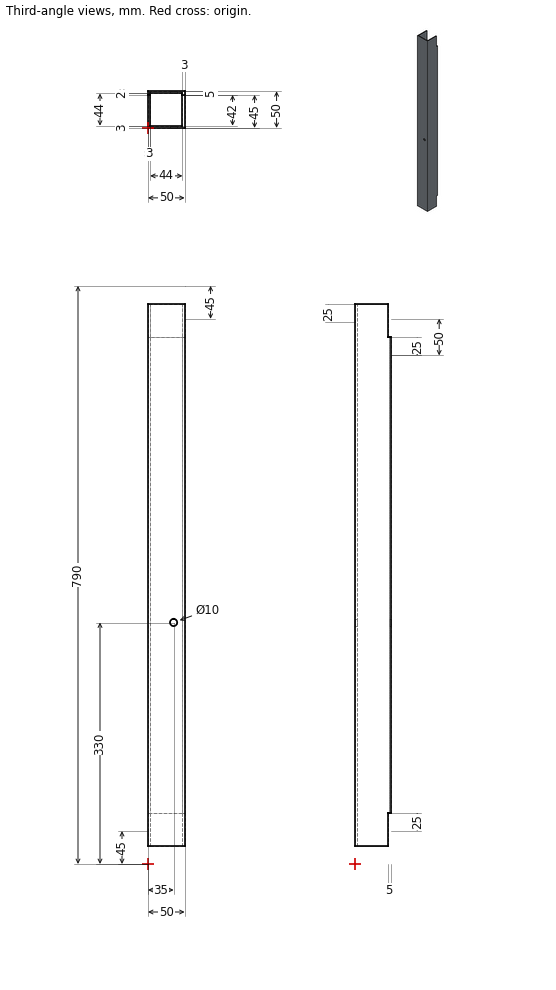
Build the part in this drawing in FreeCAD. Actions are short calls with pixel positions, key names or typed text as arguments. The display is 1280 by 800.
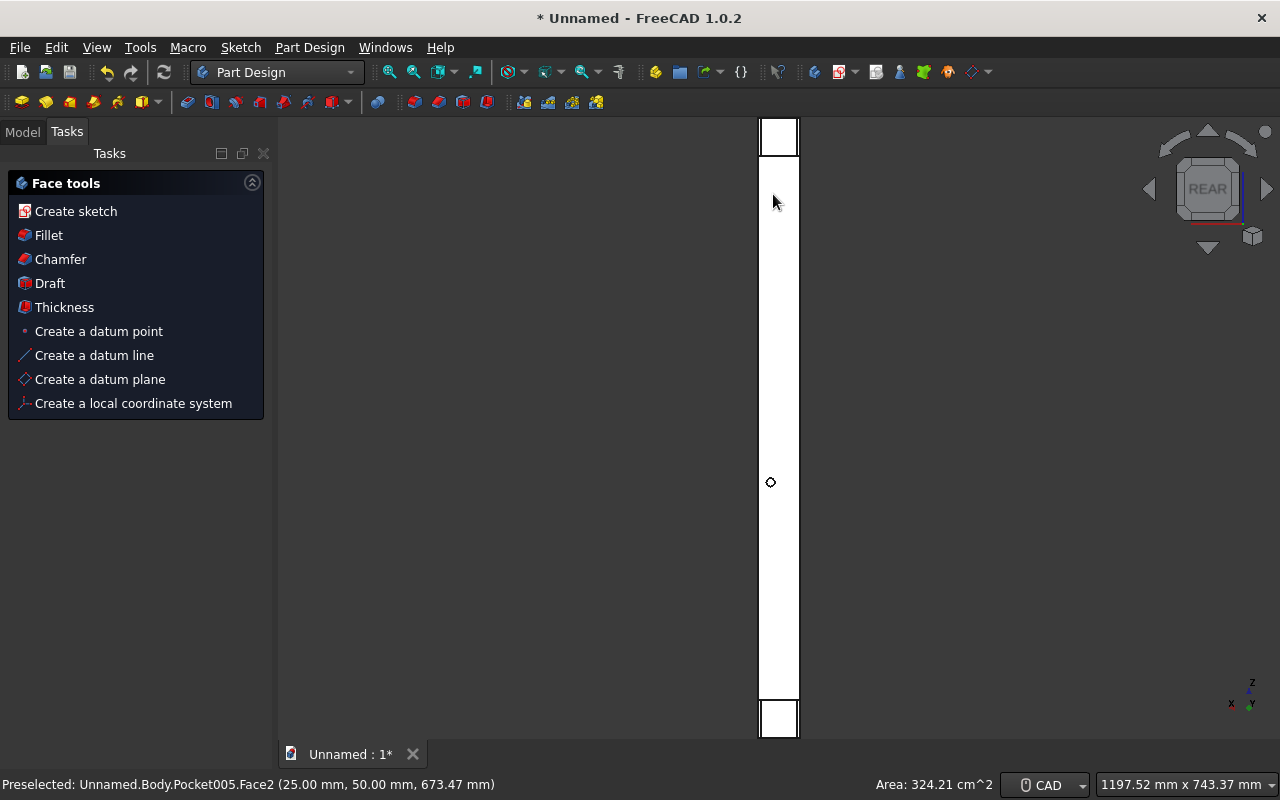
click(840, 72)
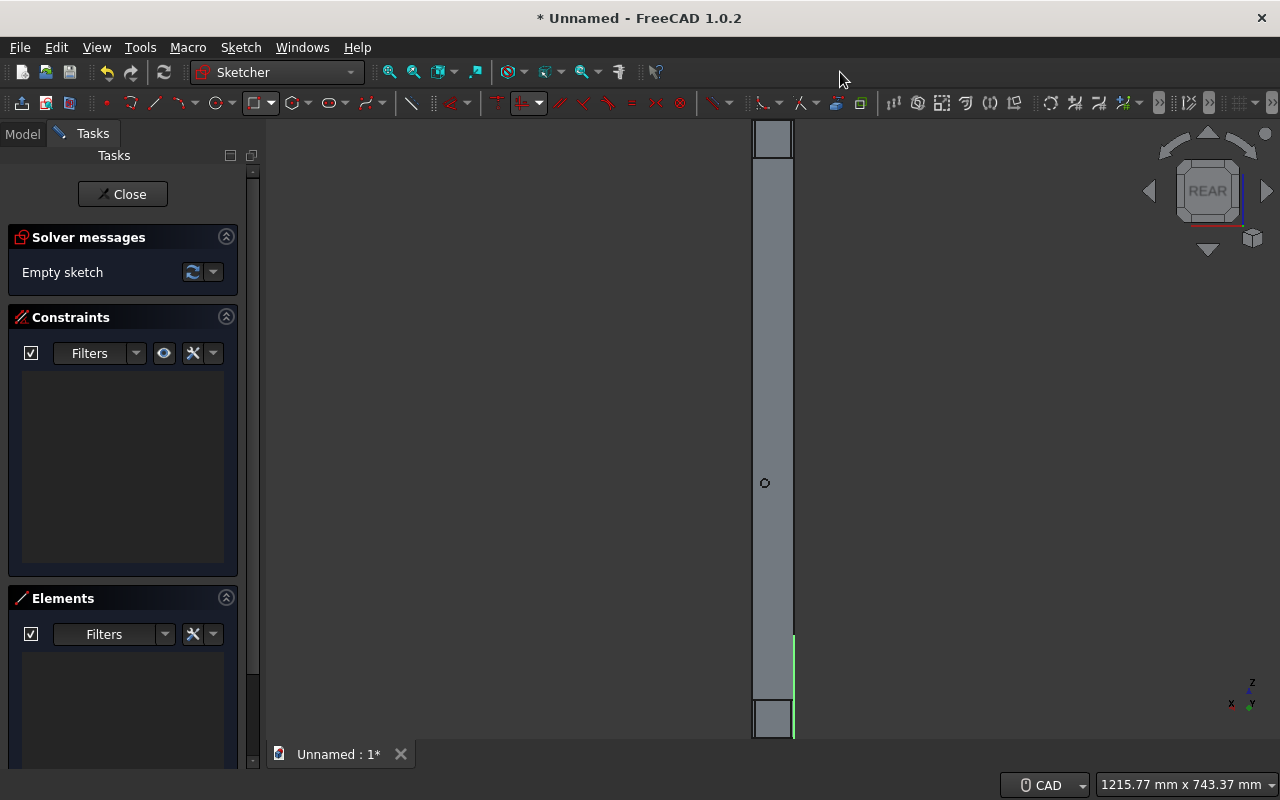
scroll(768, 486, up, 15)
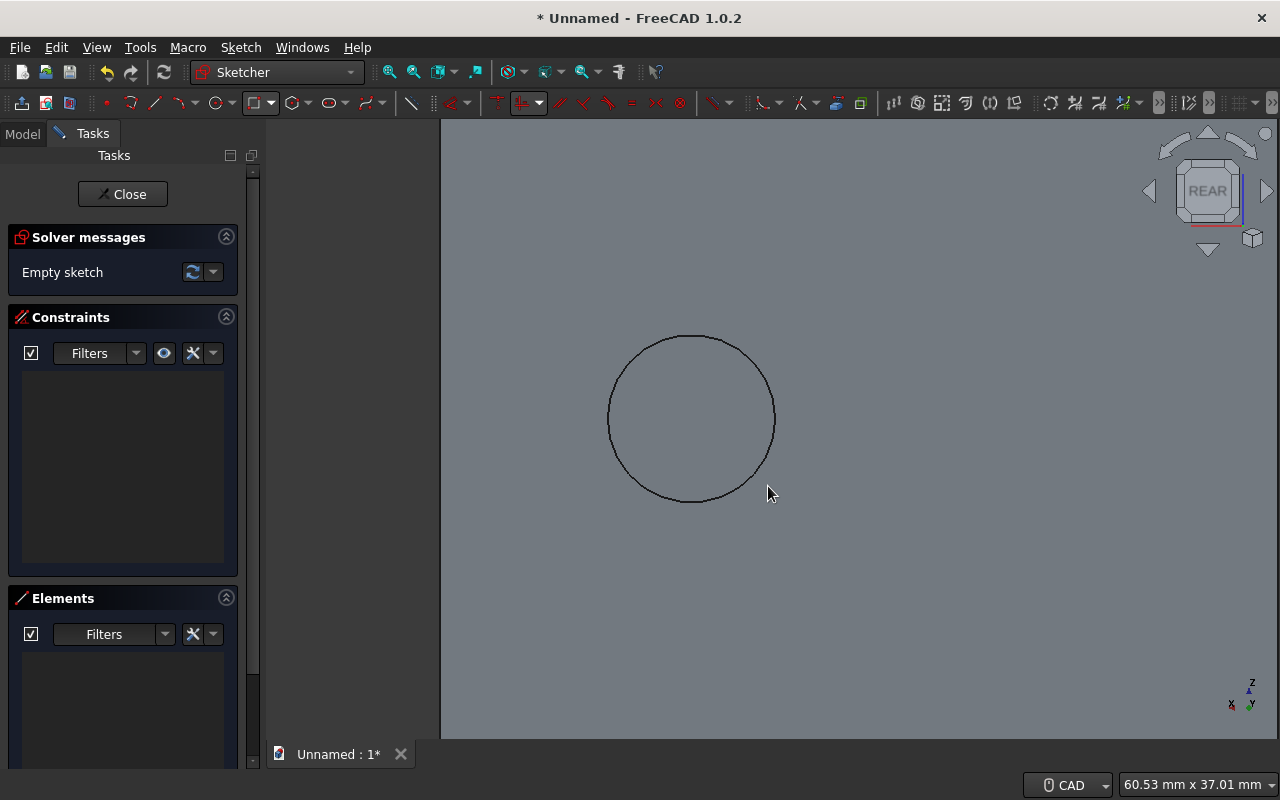
scroll(681, 410, up, 4)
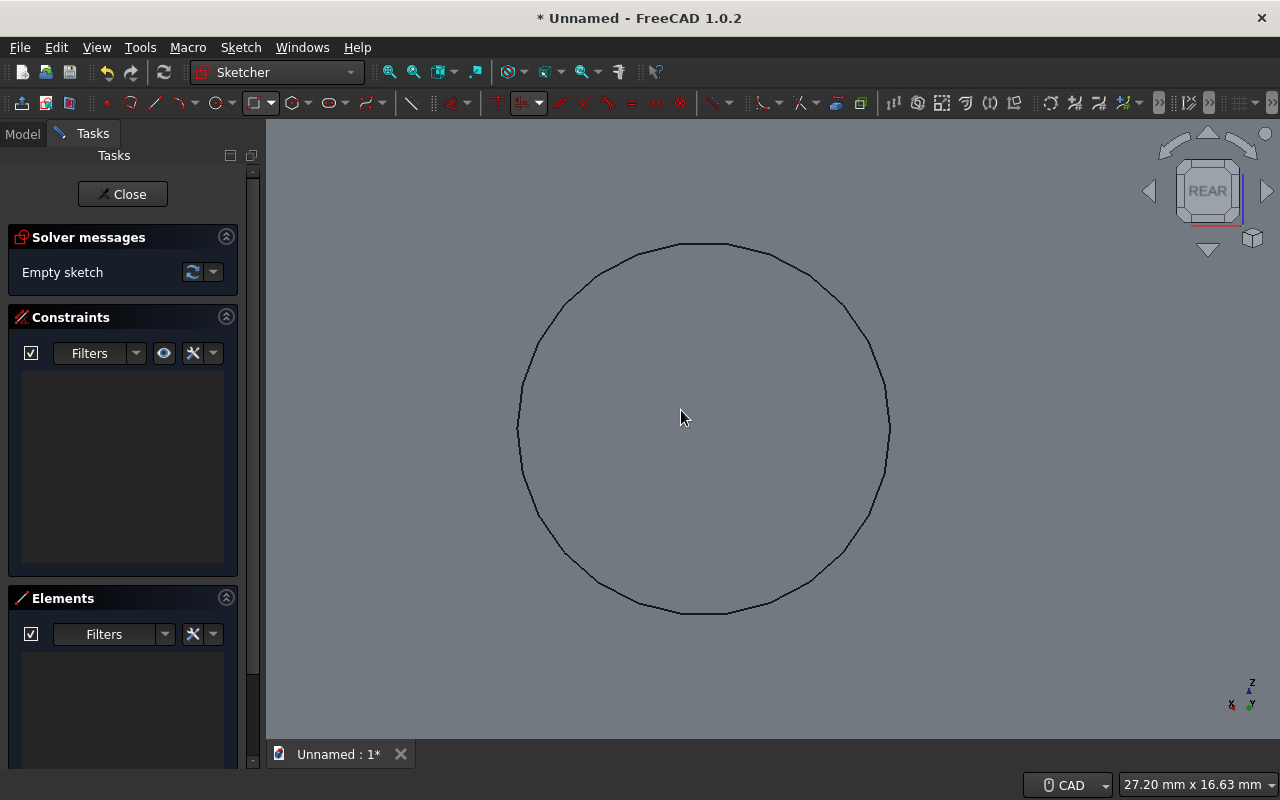
click(216, 104)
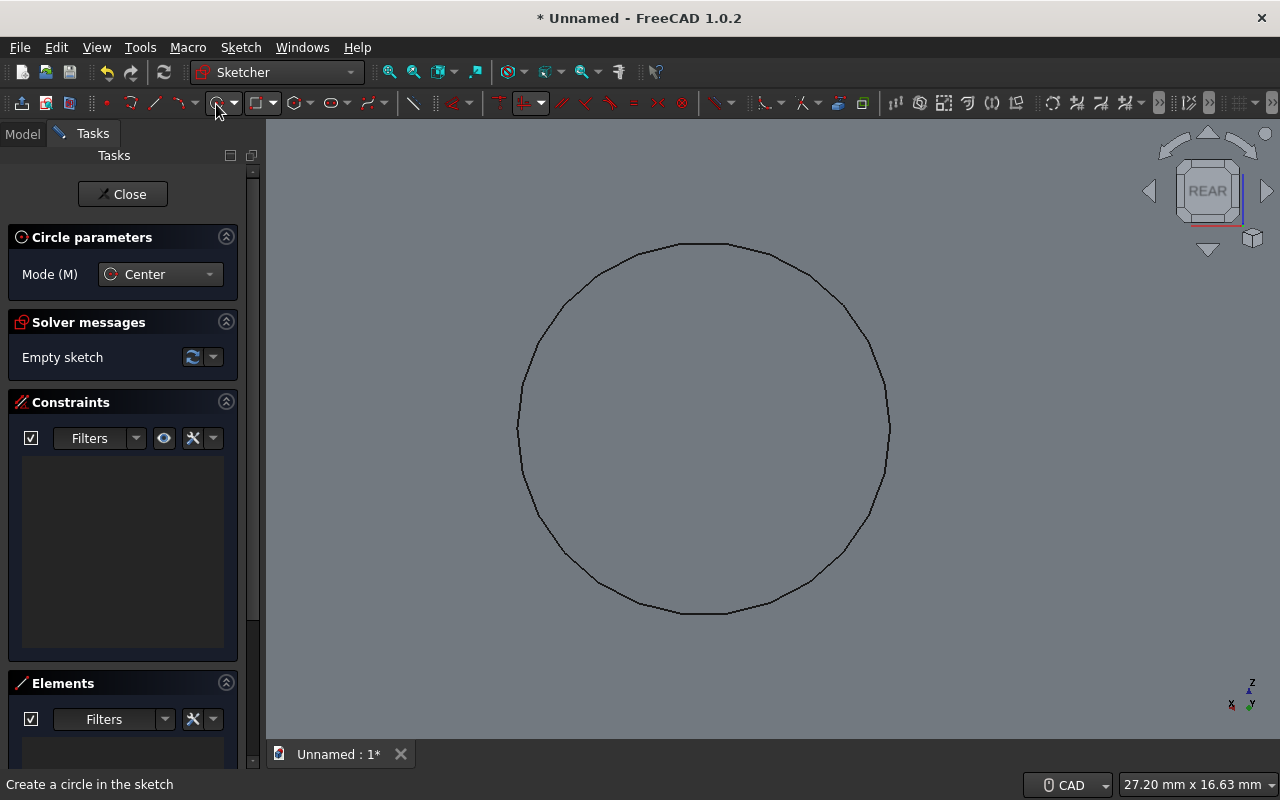
click(704, 429)
click(836, 297)
key(Escape)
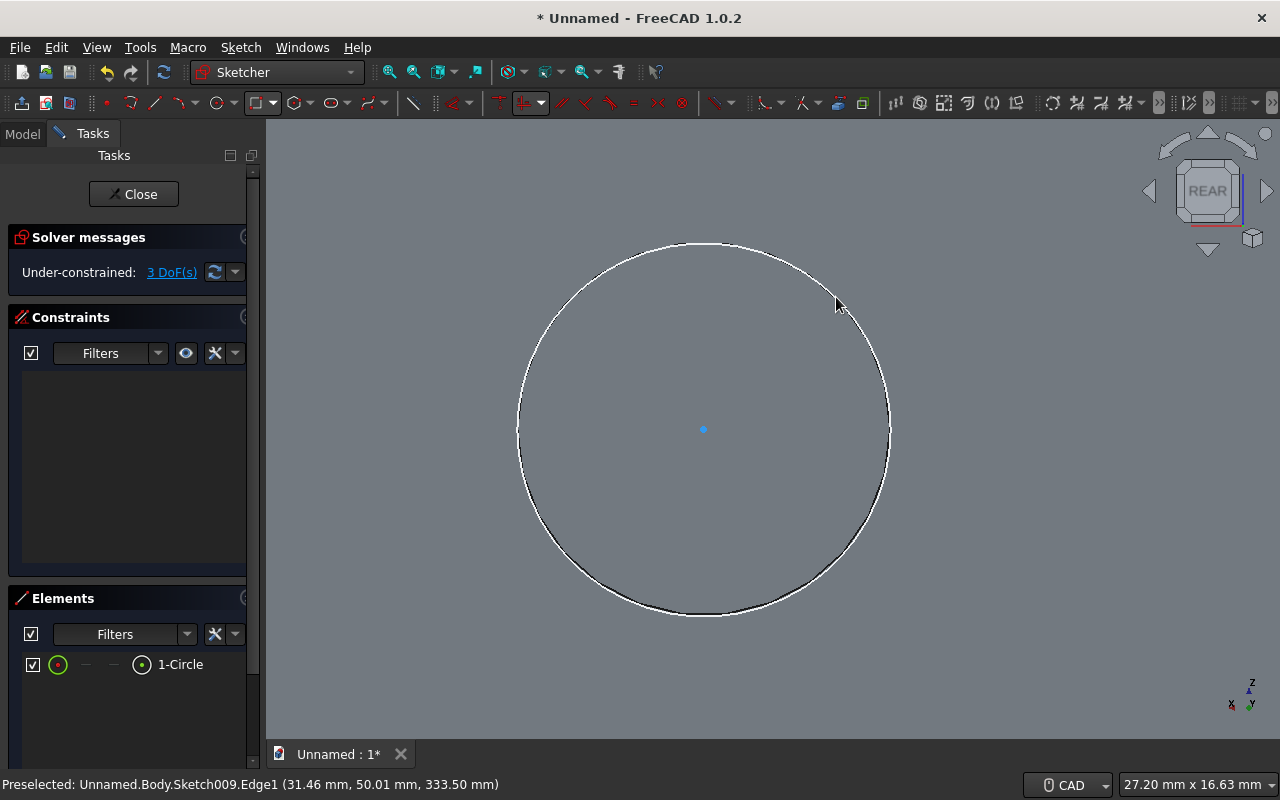
click(452, 104)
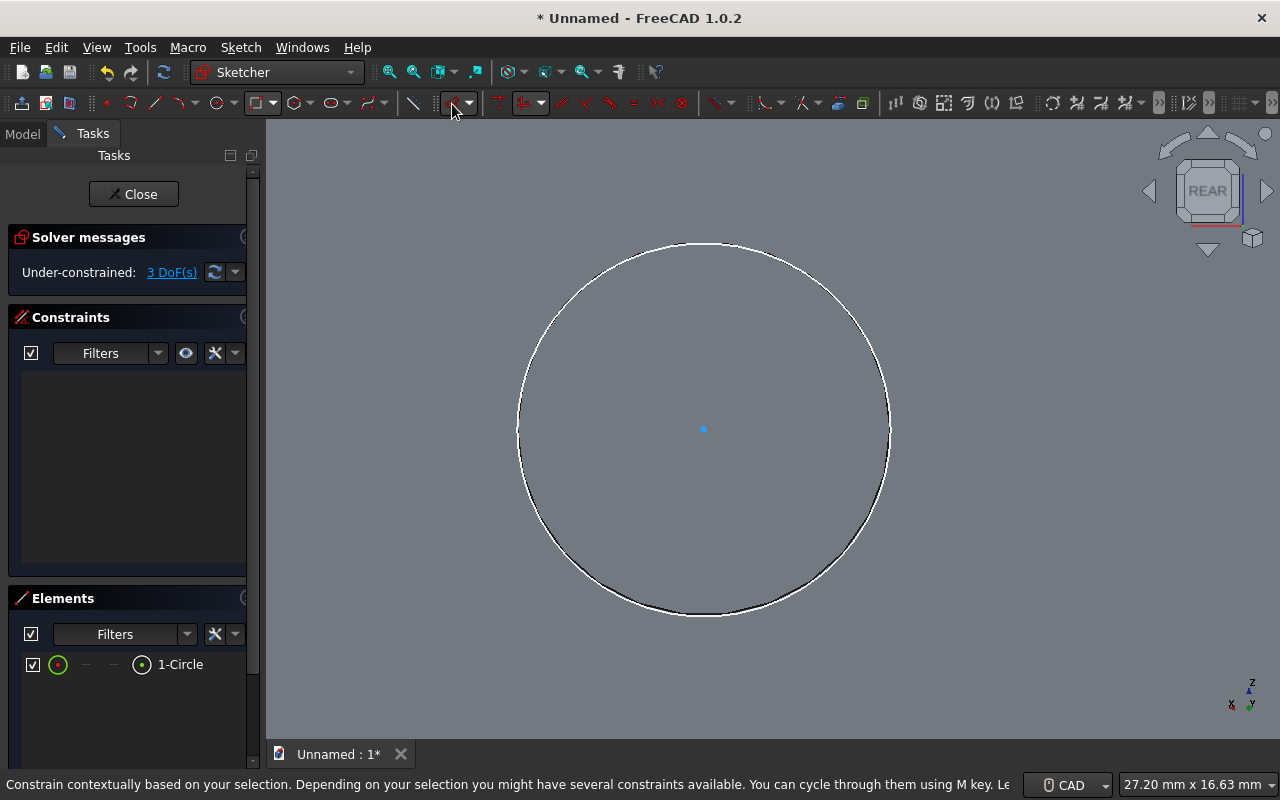
click(836, 298)
click(859, 275)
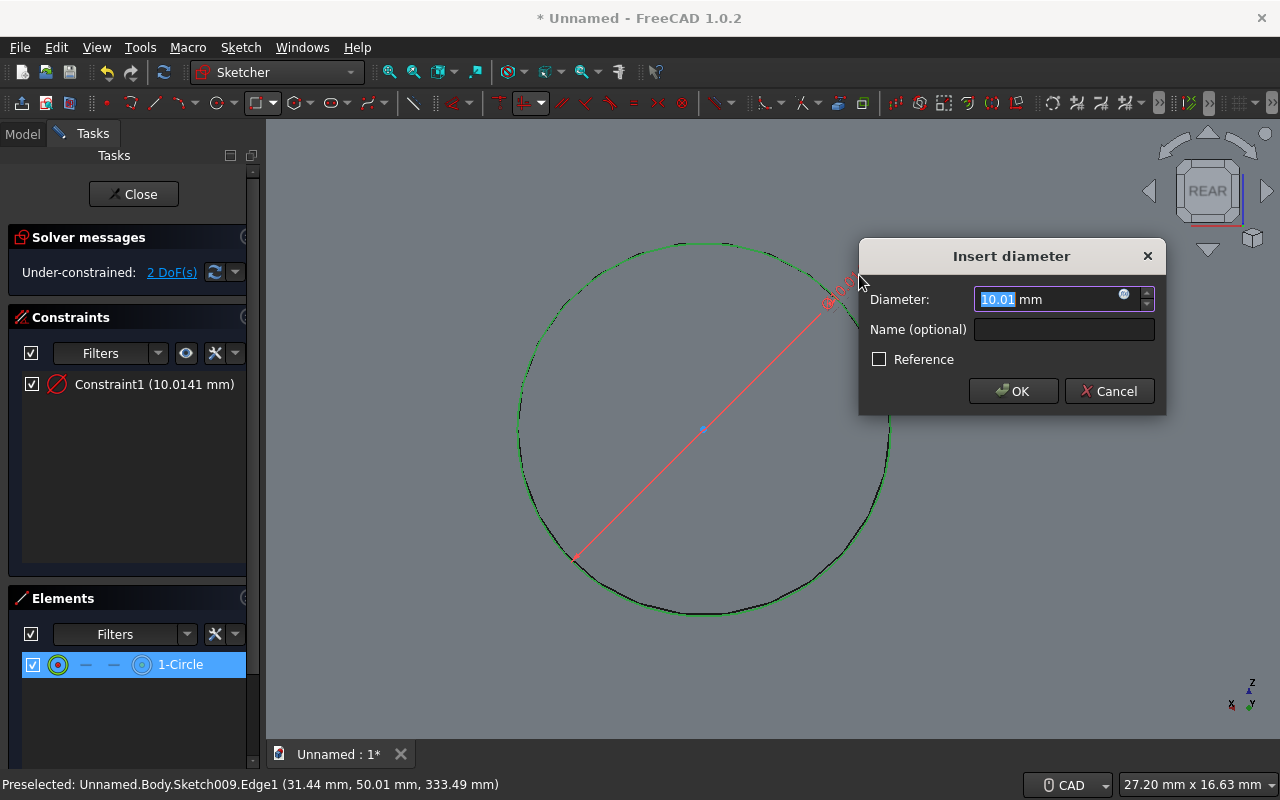
text(10)
key(Return)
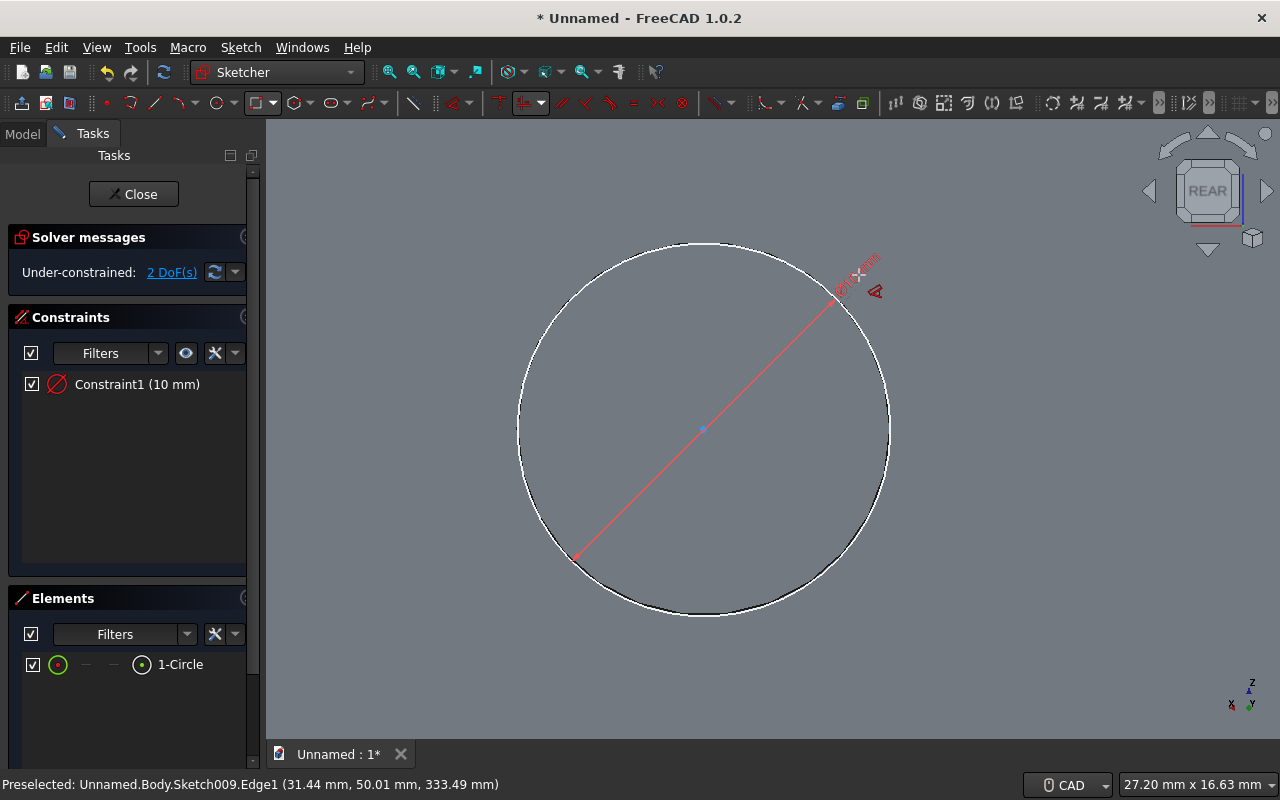
click(704, 430)
click(909, 396)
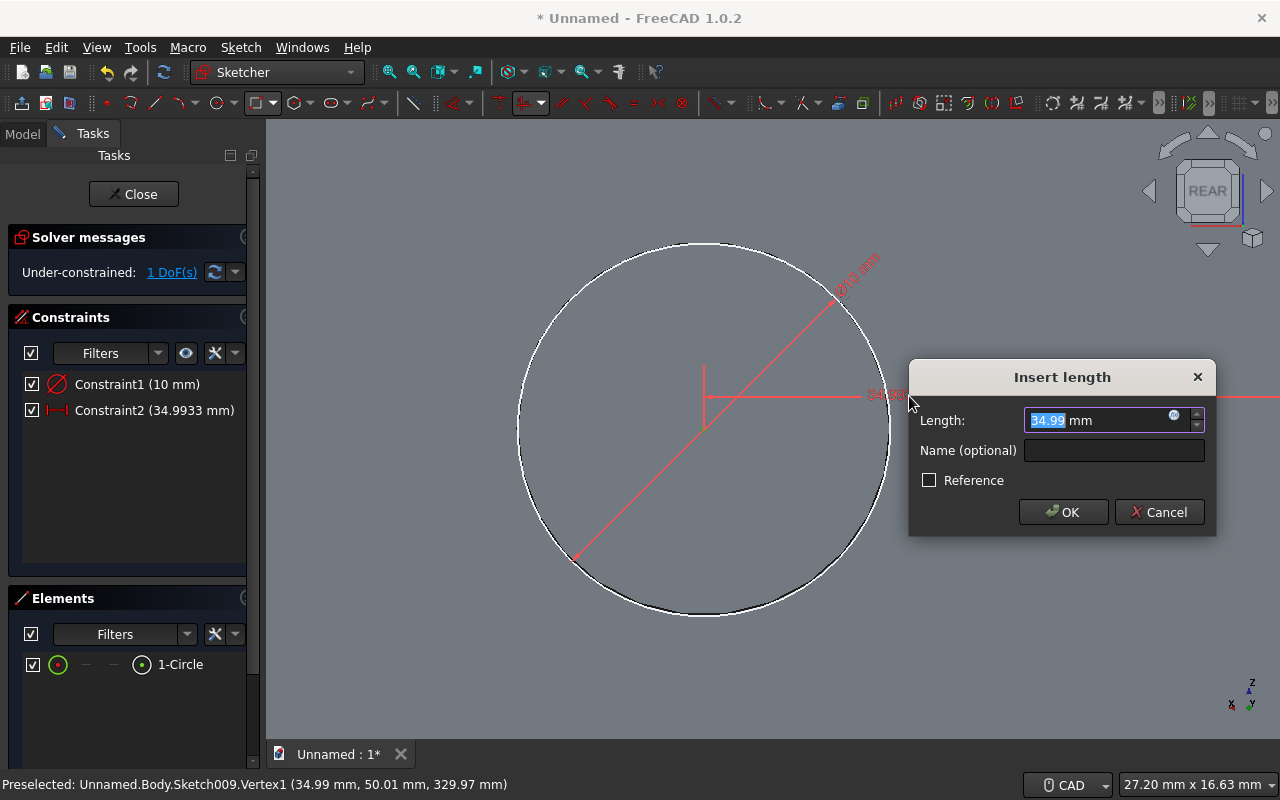
text(35)
key(Return)